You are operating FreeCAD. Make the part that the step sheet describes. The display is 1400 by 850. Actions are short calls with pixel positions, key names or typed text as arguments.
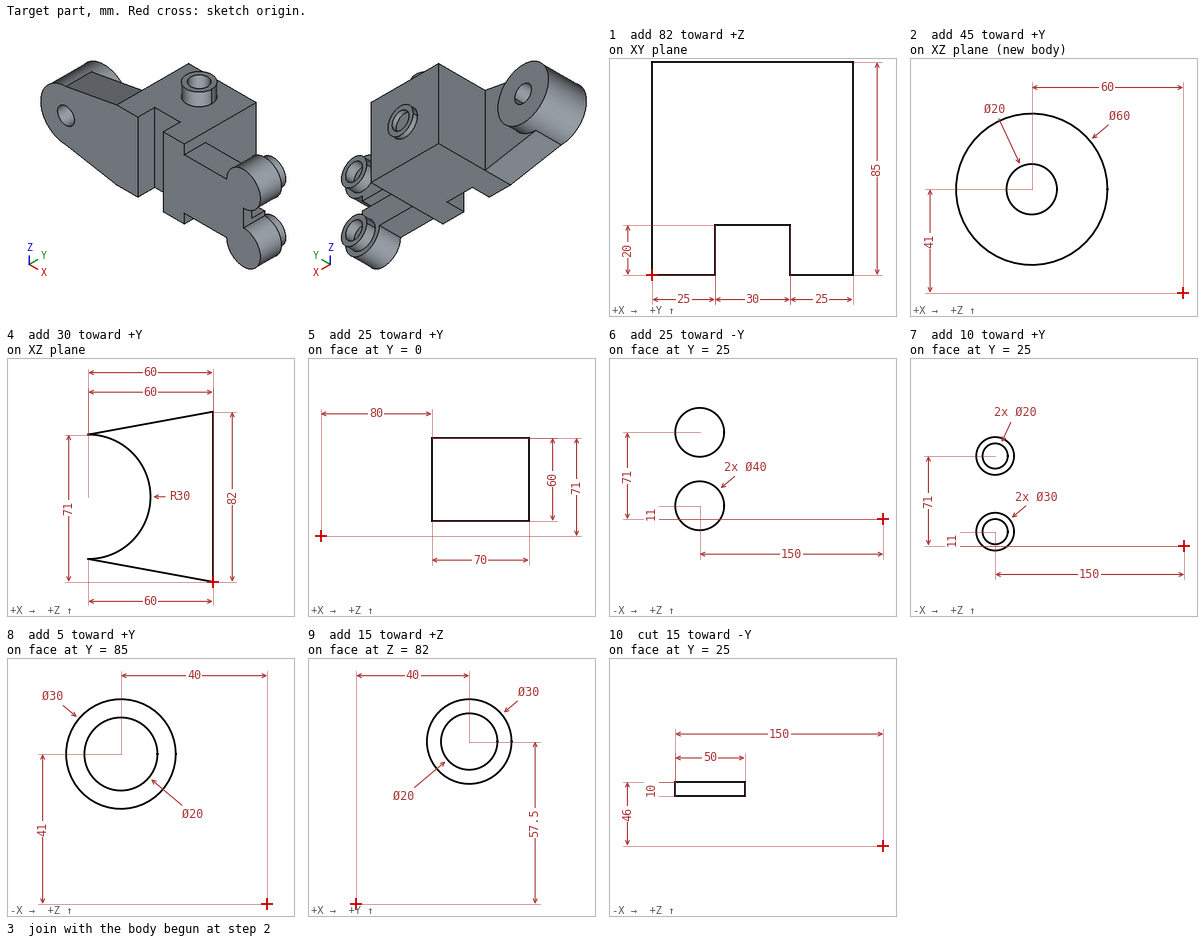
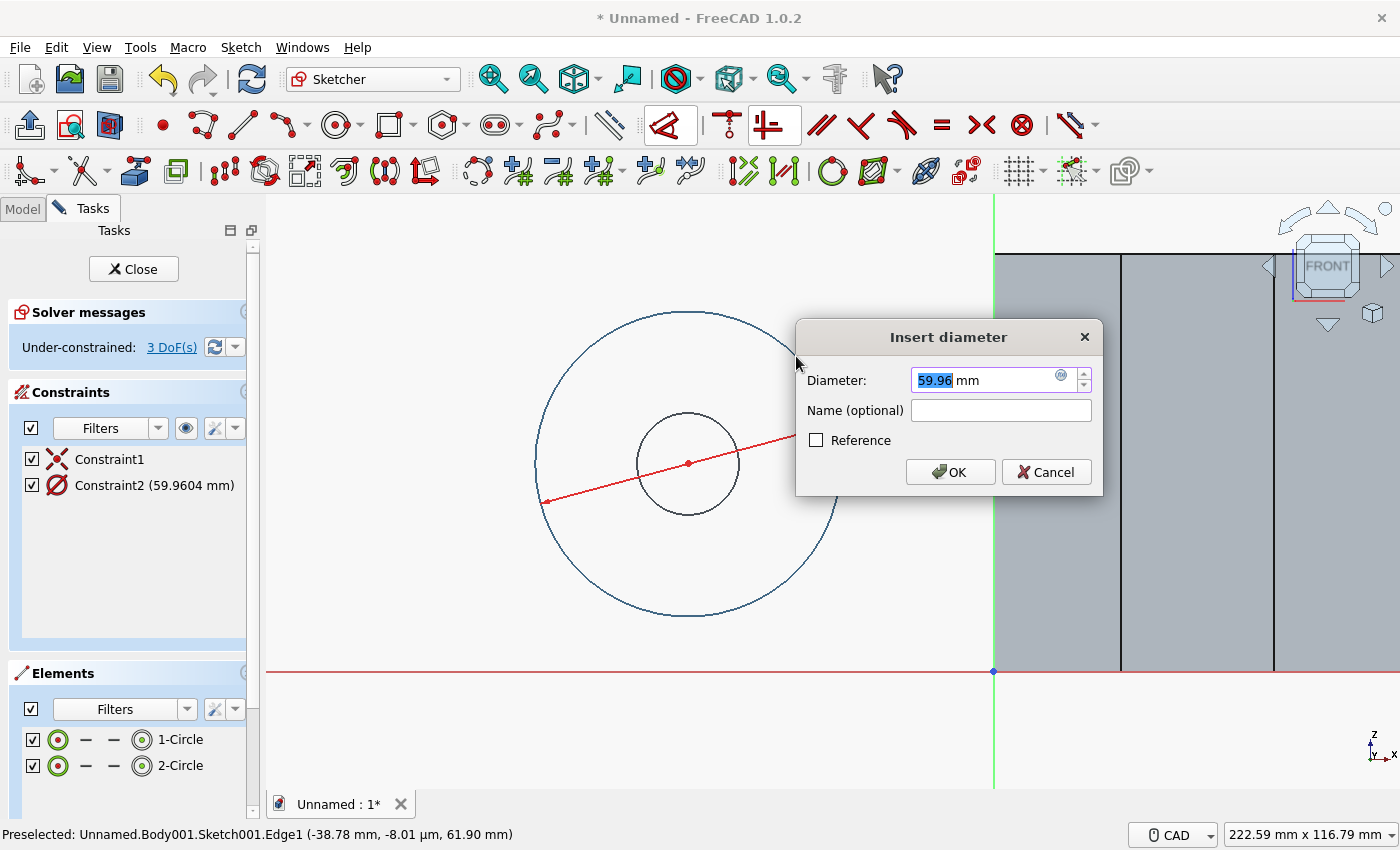
text(60)
key(Return)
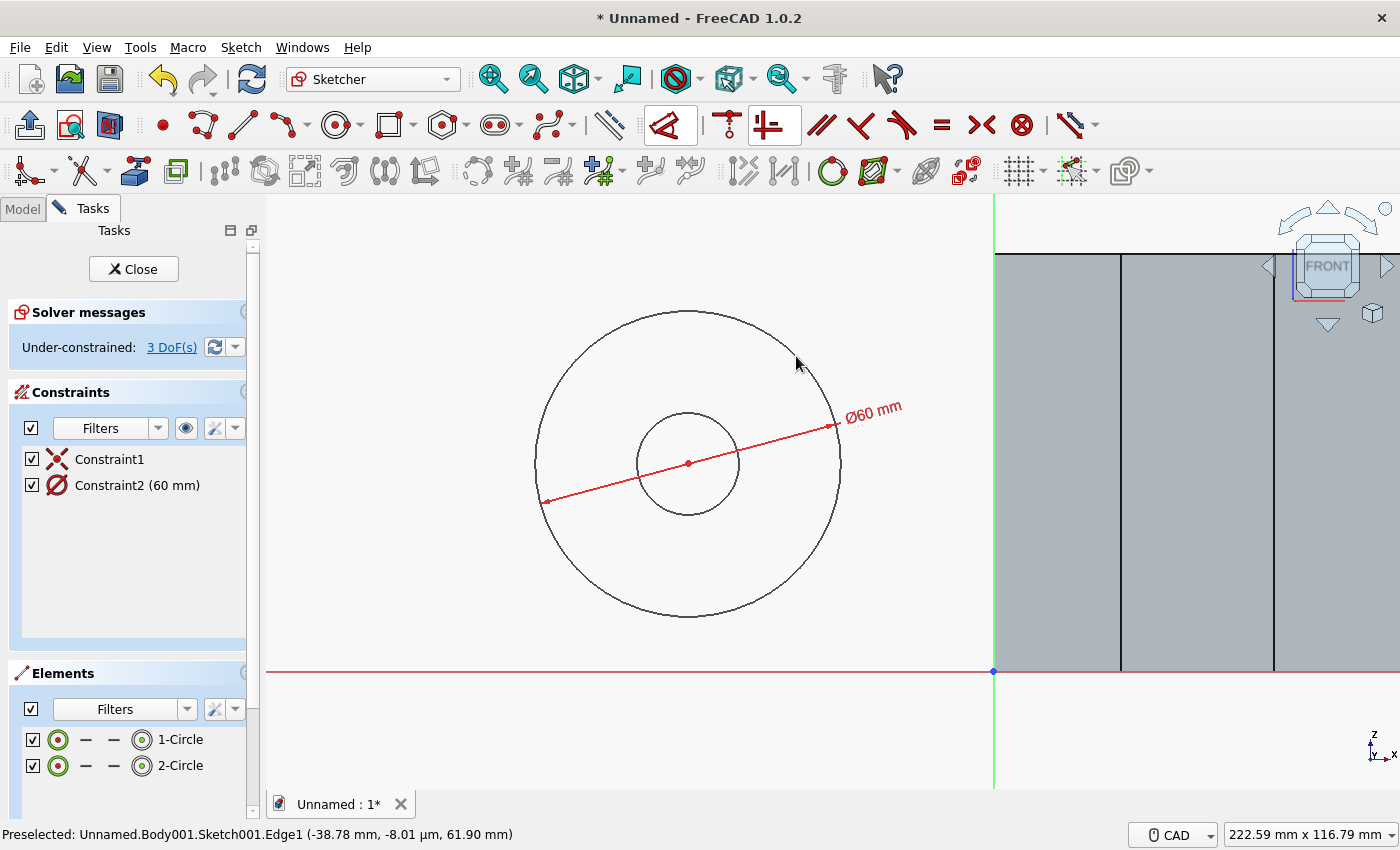
click(724, 428)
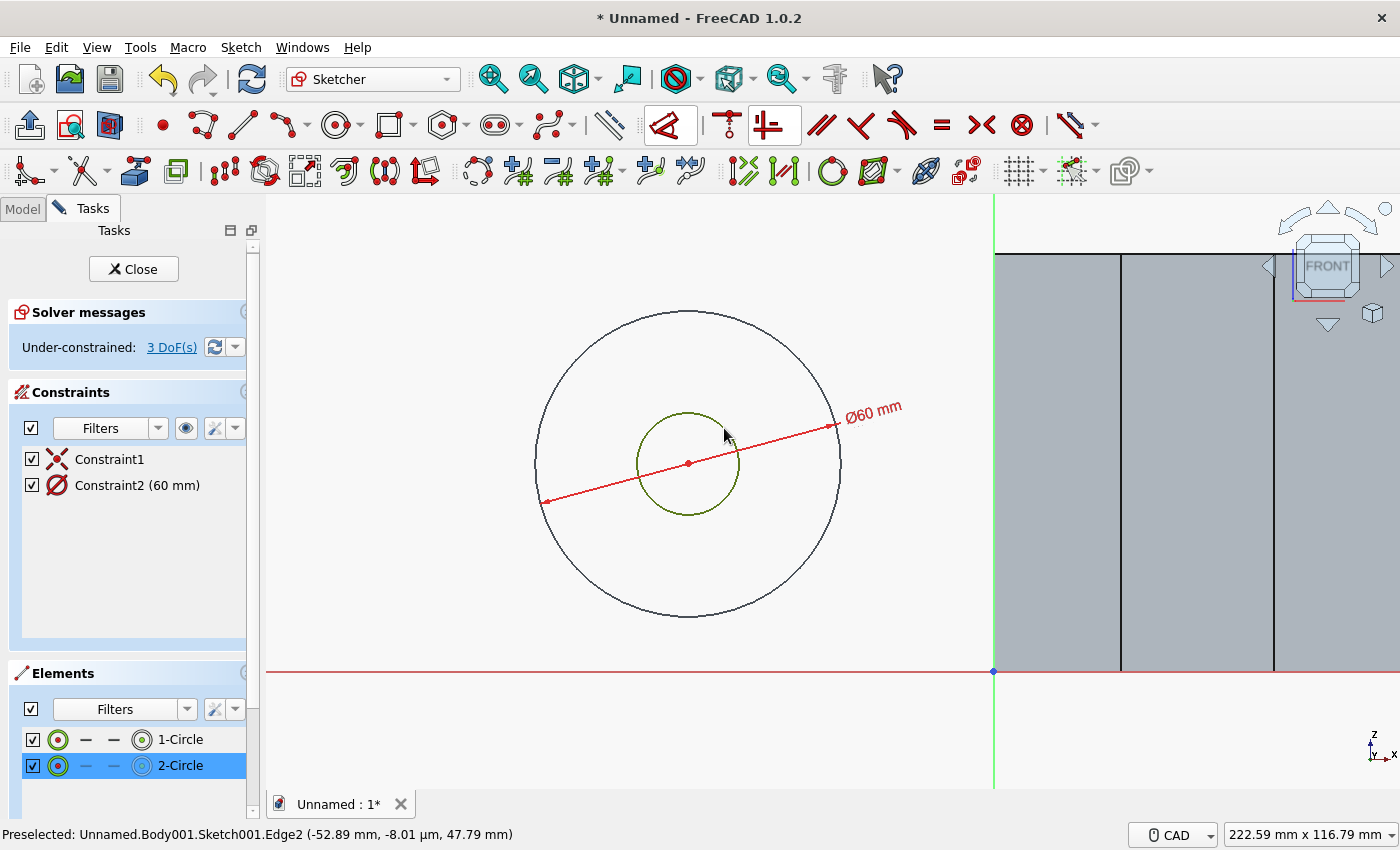
key(k)
key(o)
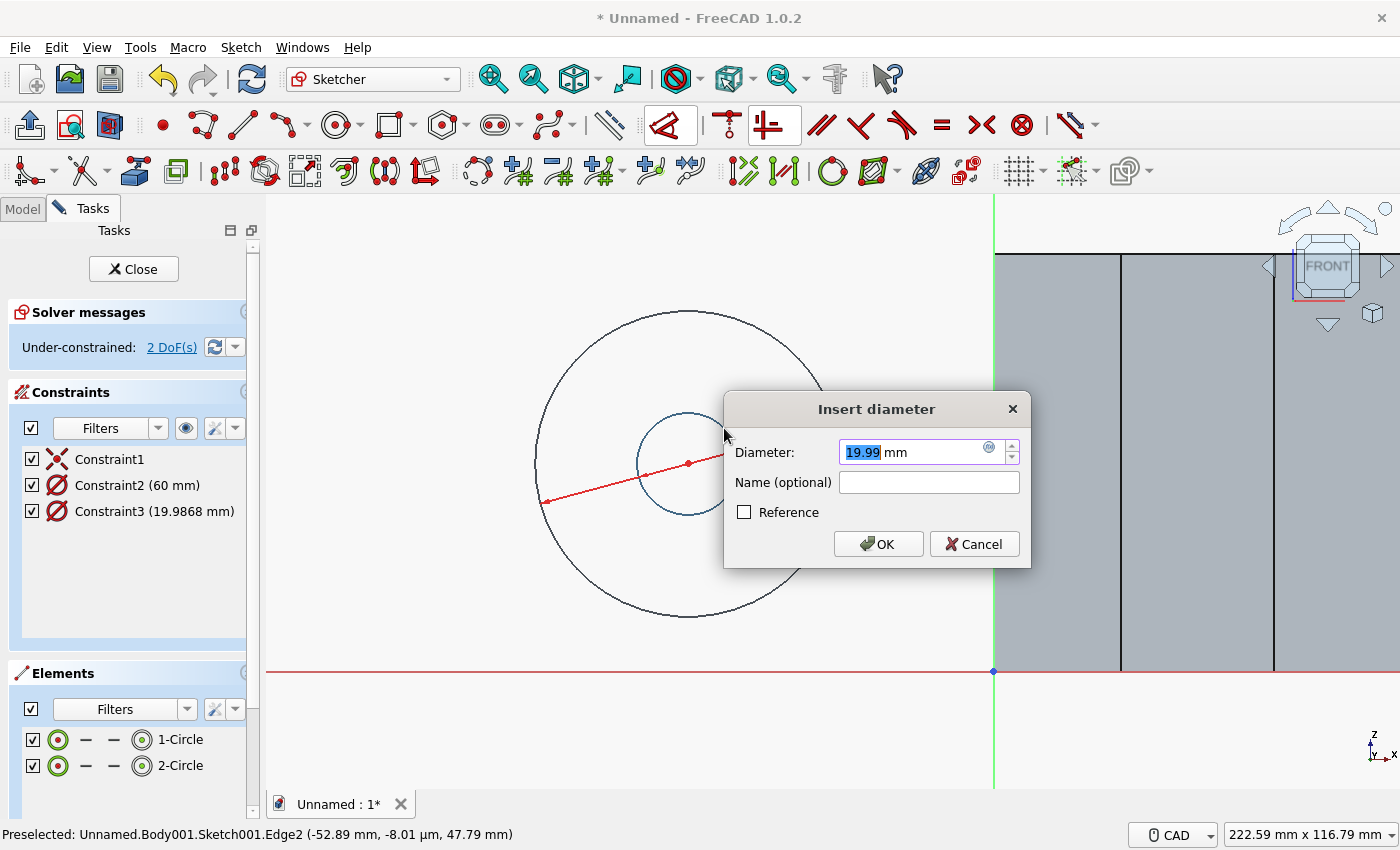
text(20)
key(Return)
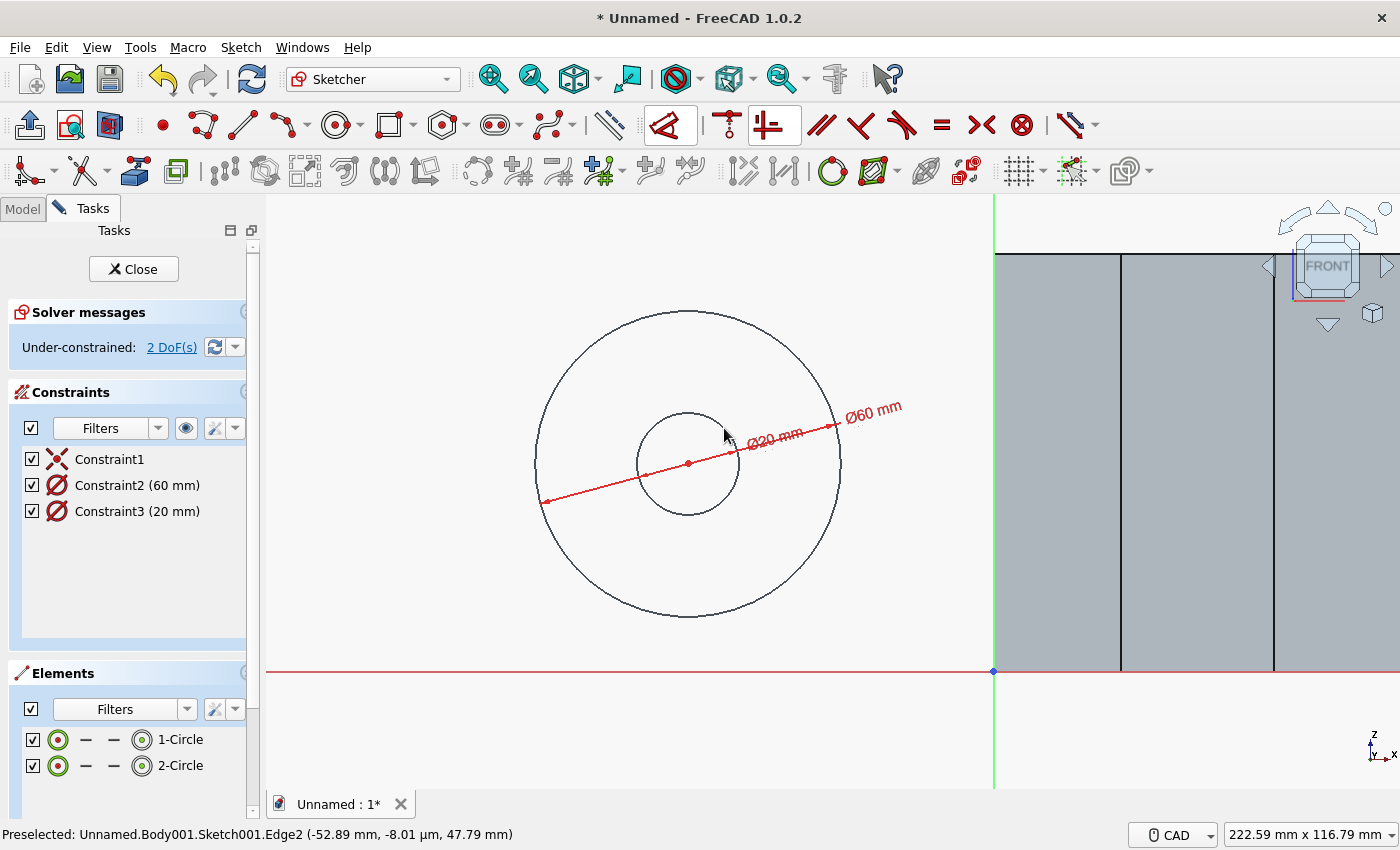
click(688, 464)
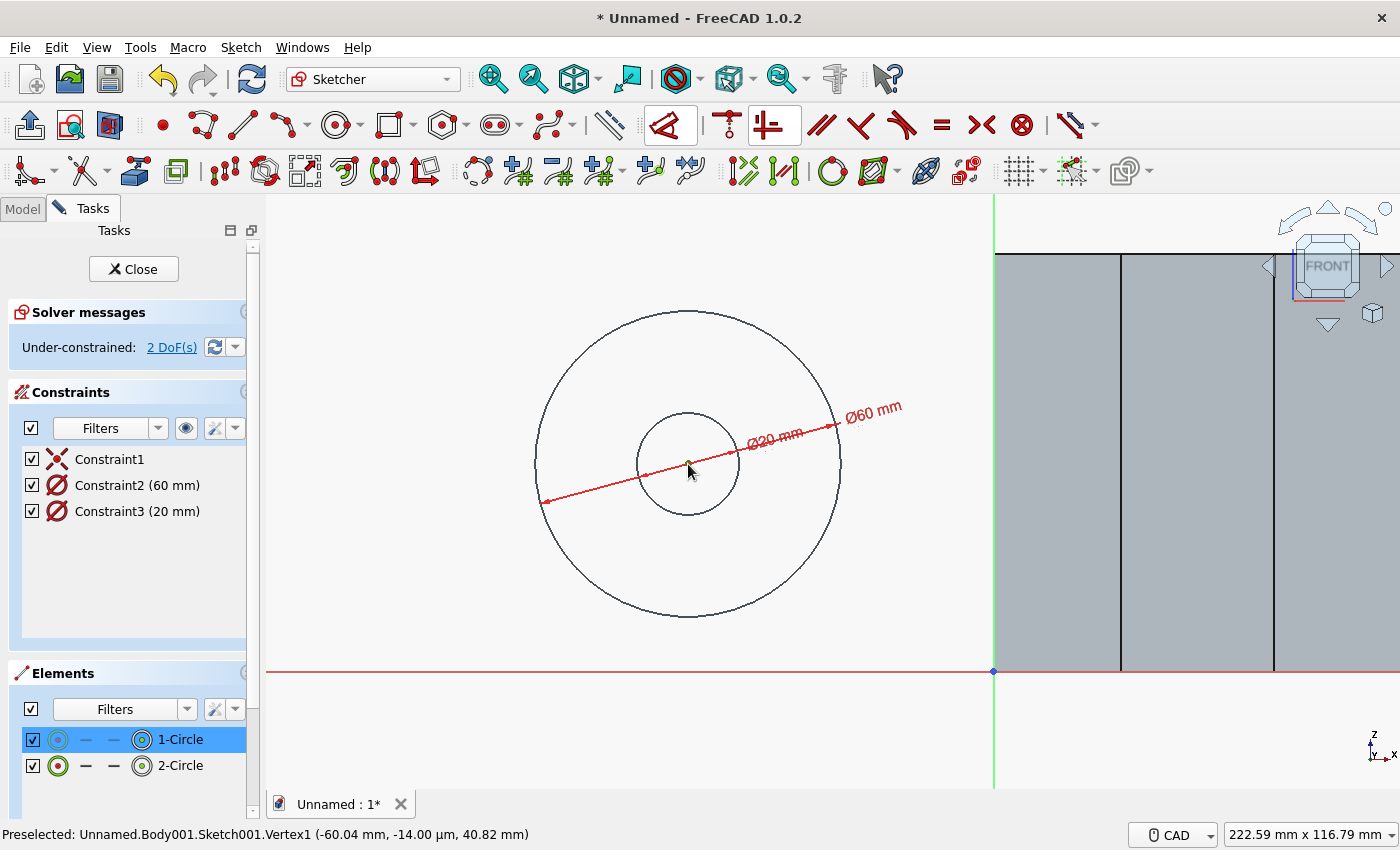
click(692, 126)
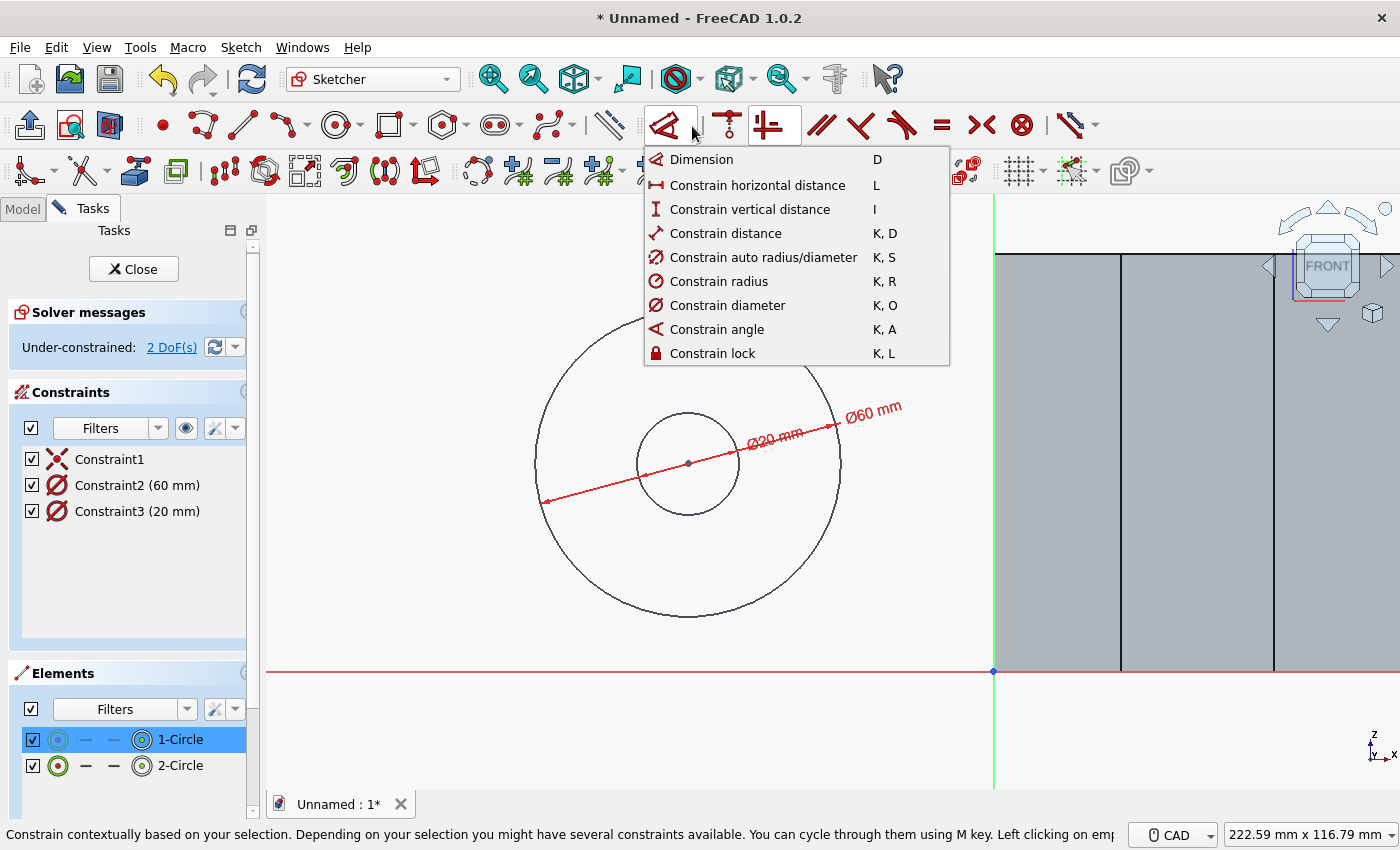
click(797, 185)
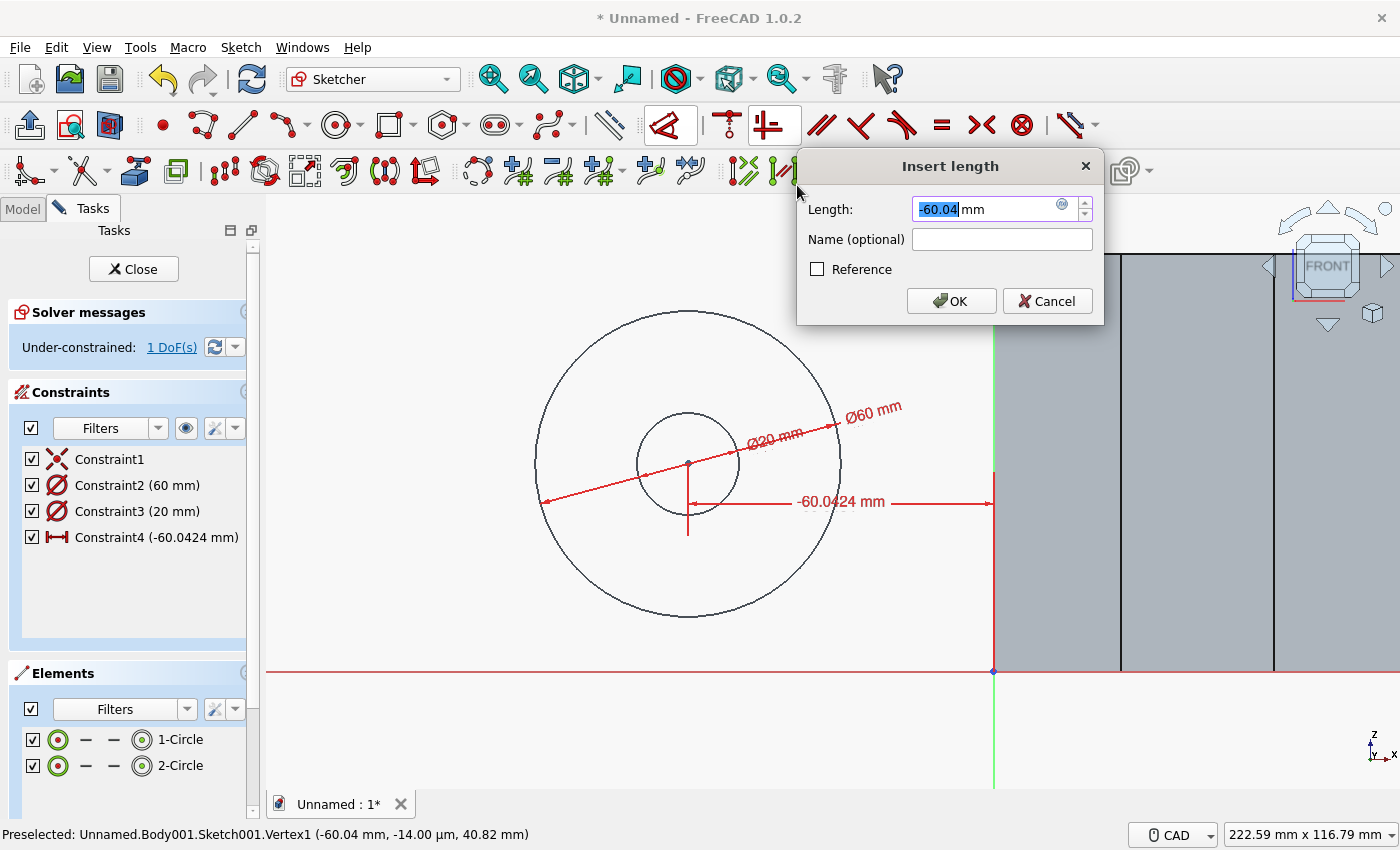
text(-60)
key(Return)